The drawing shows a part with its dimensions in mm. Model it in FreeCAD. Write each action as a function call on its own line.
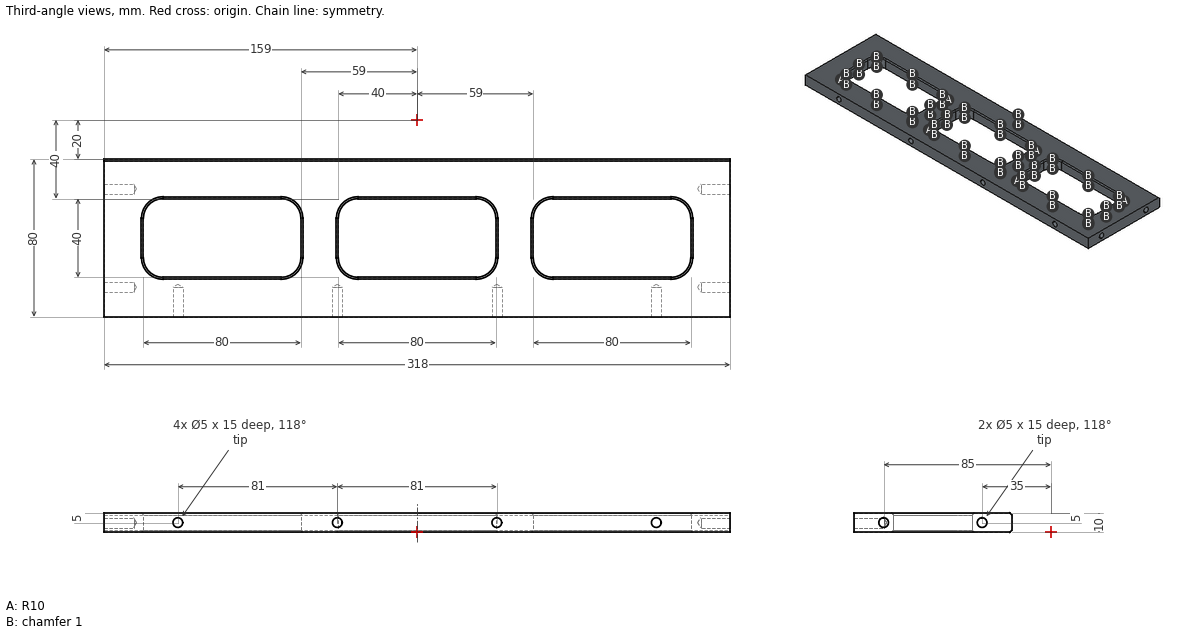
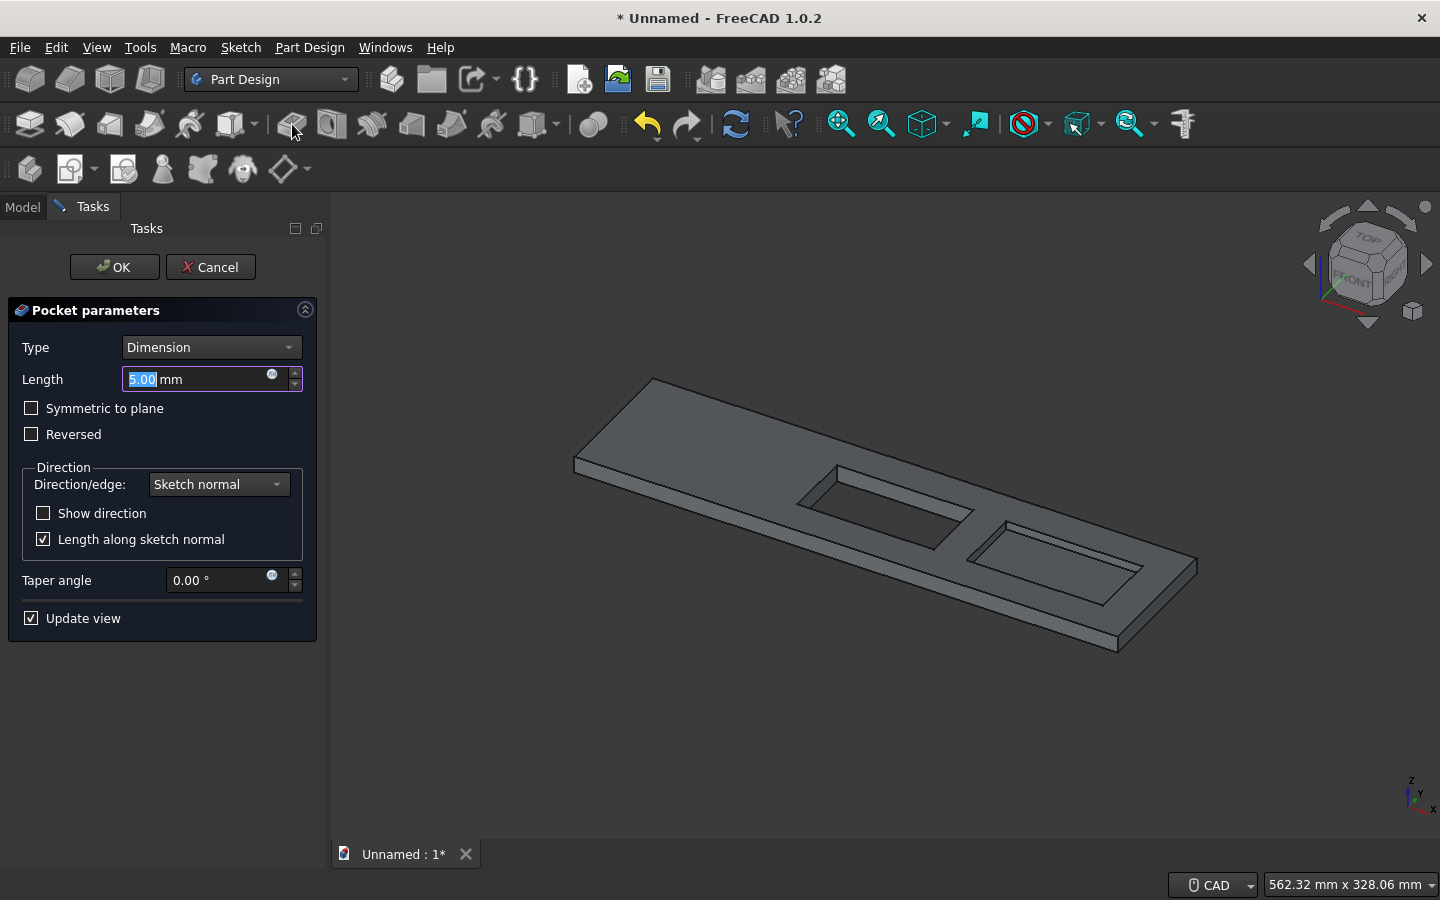
click(212, 348)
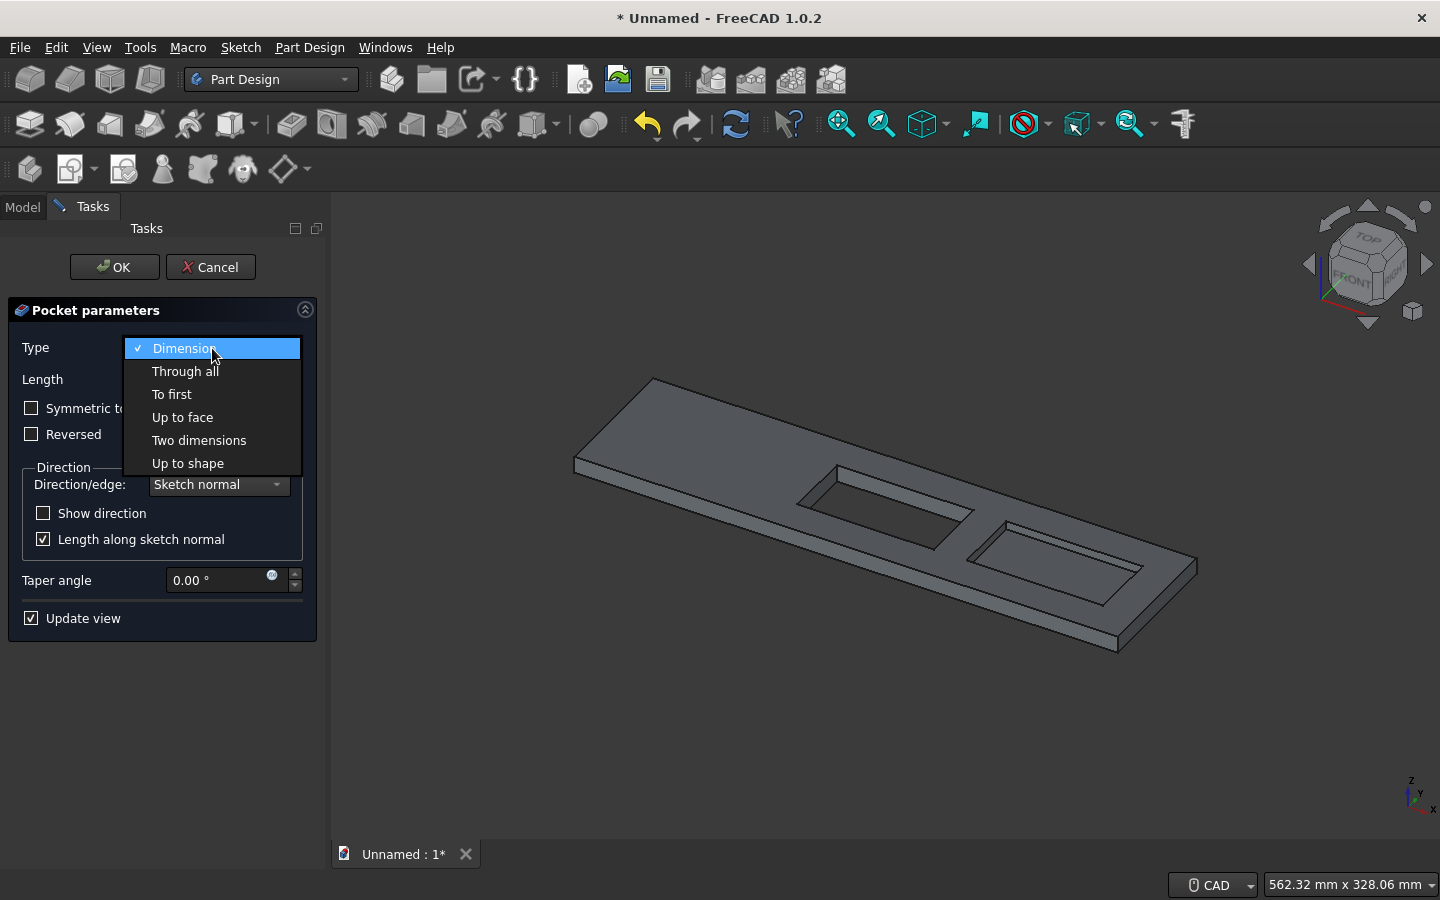
click(212, 372)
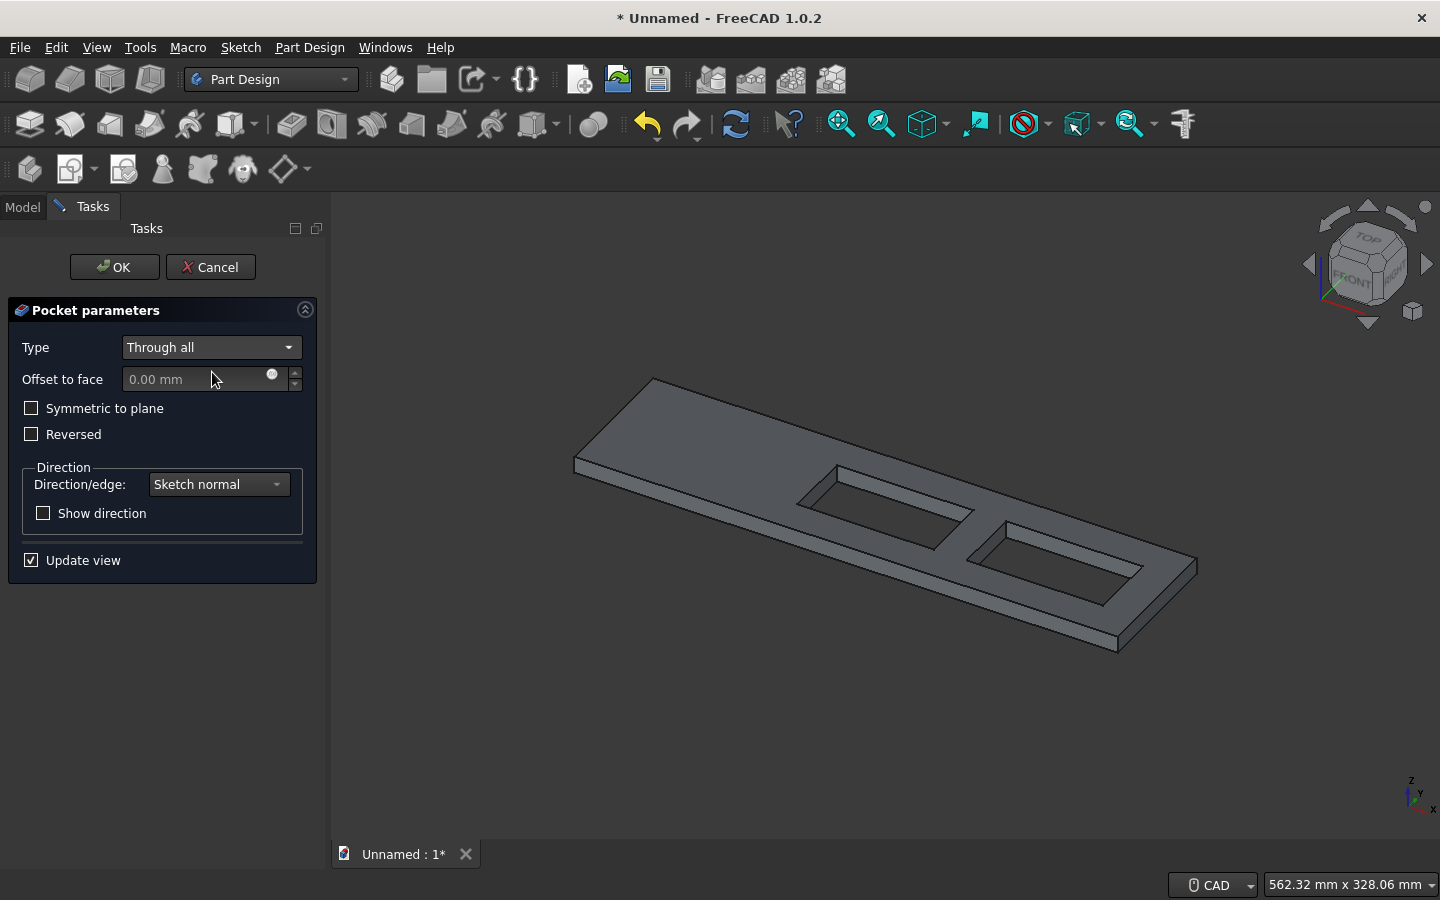
click(115, 267)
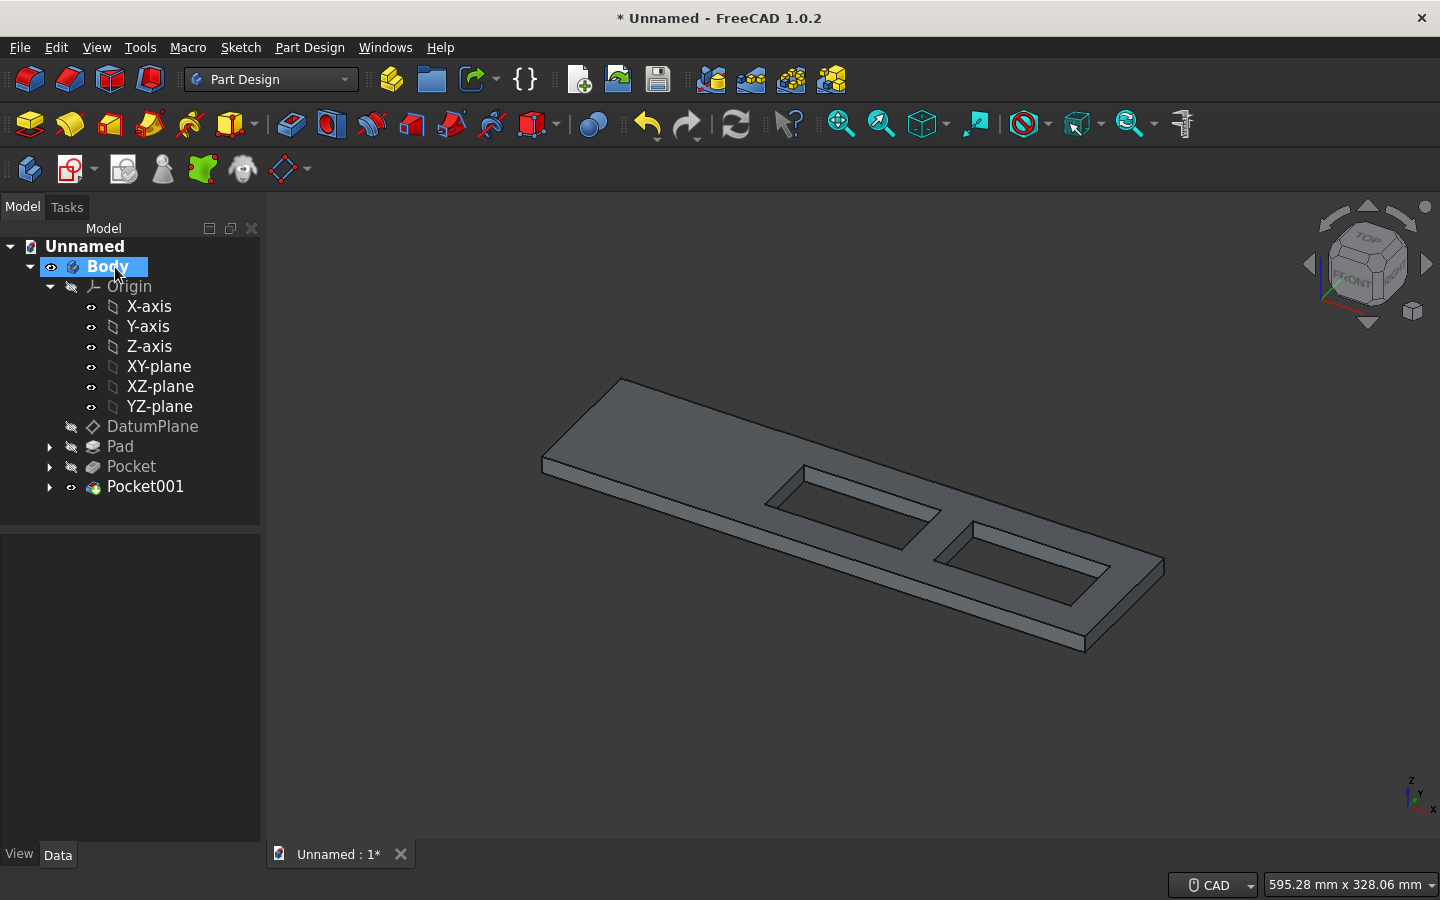
click(70, 170)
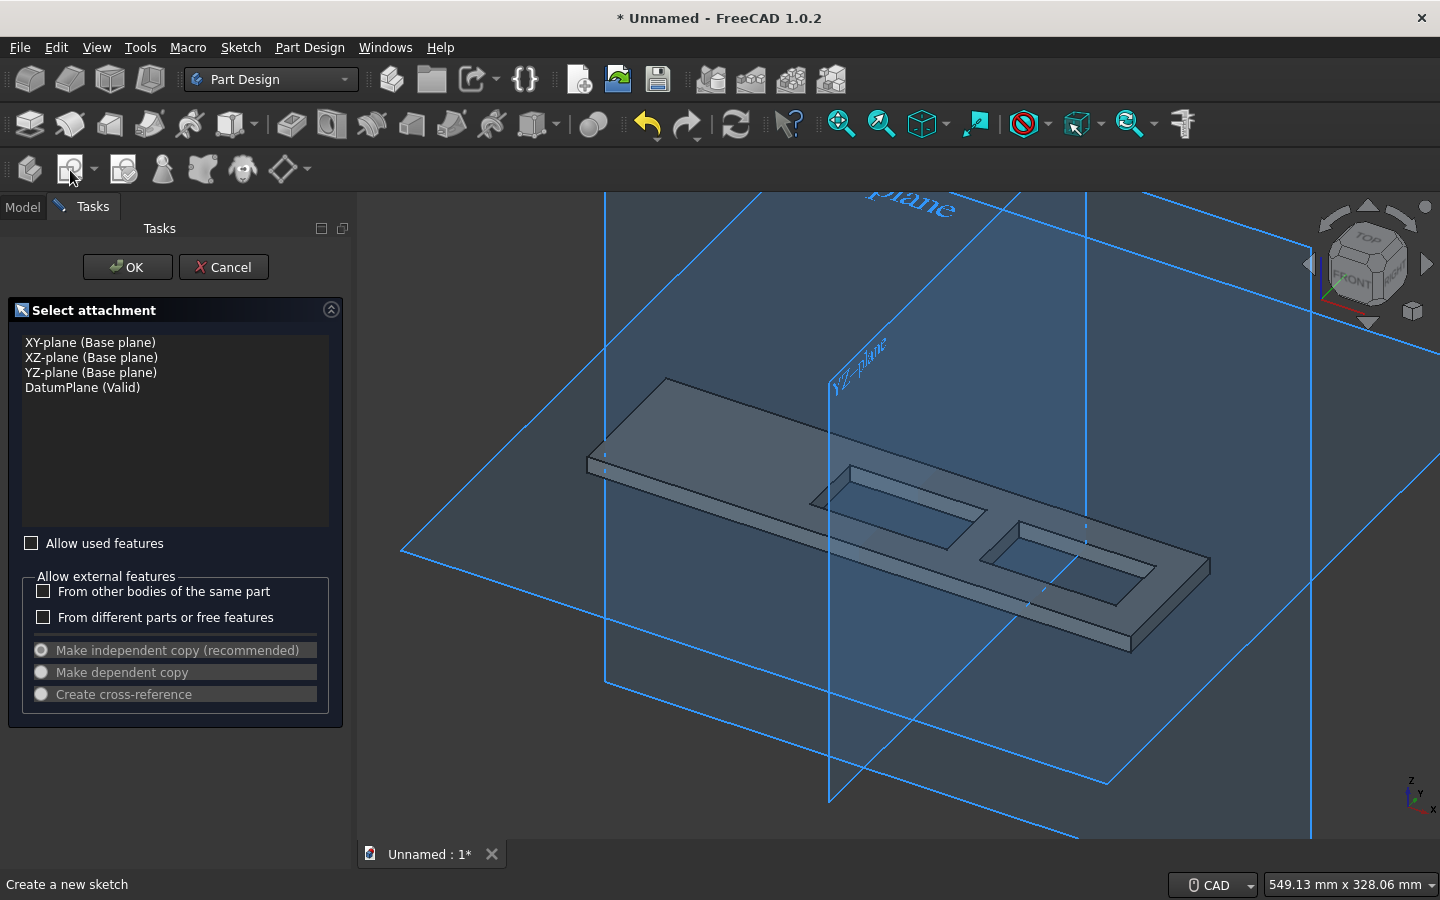
click(82, 342)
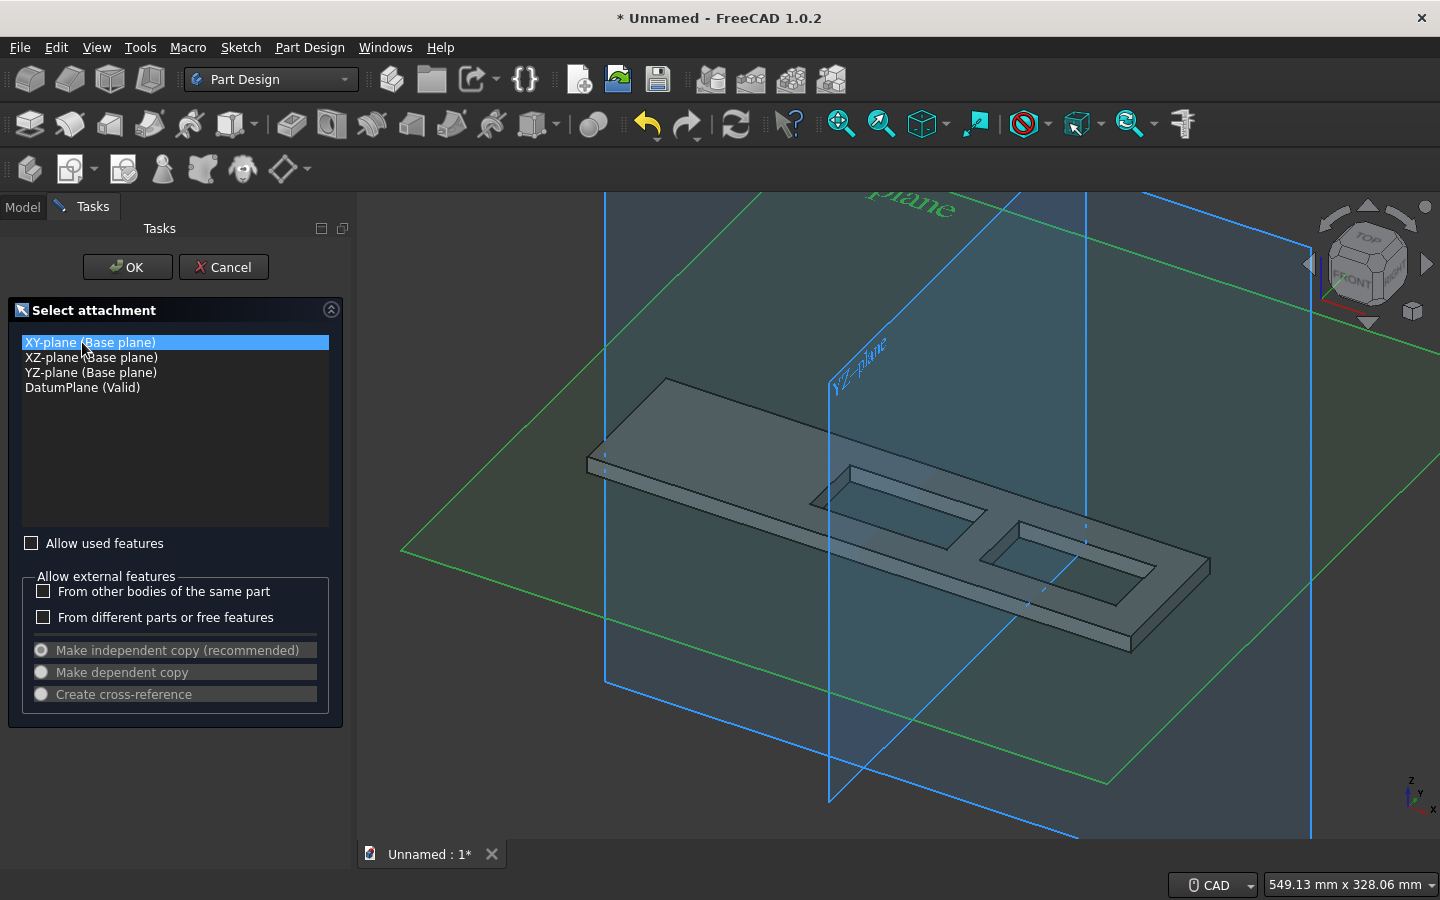
click(128, 267)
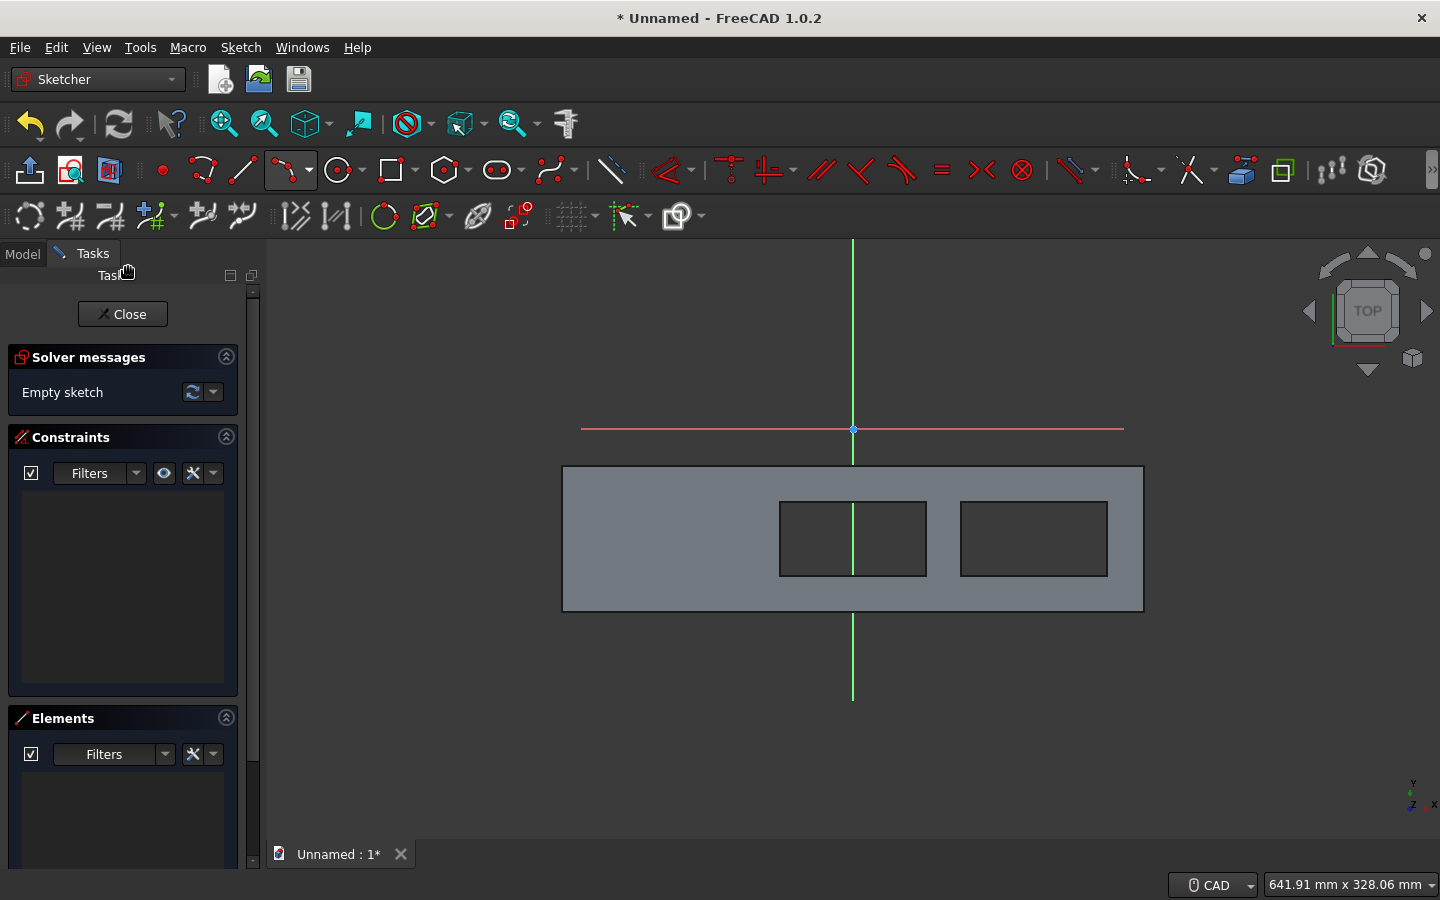
click(110, 170)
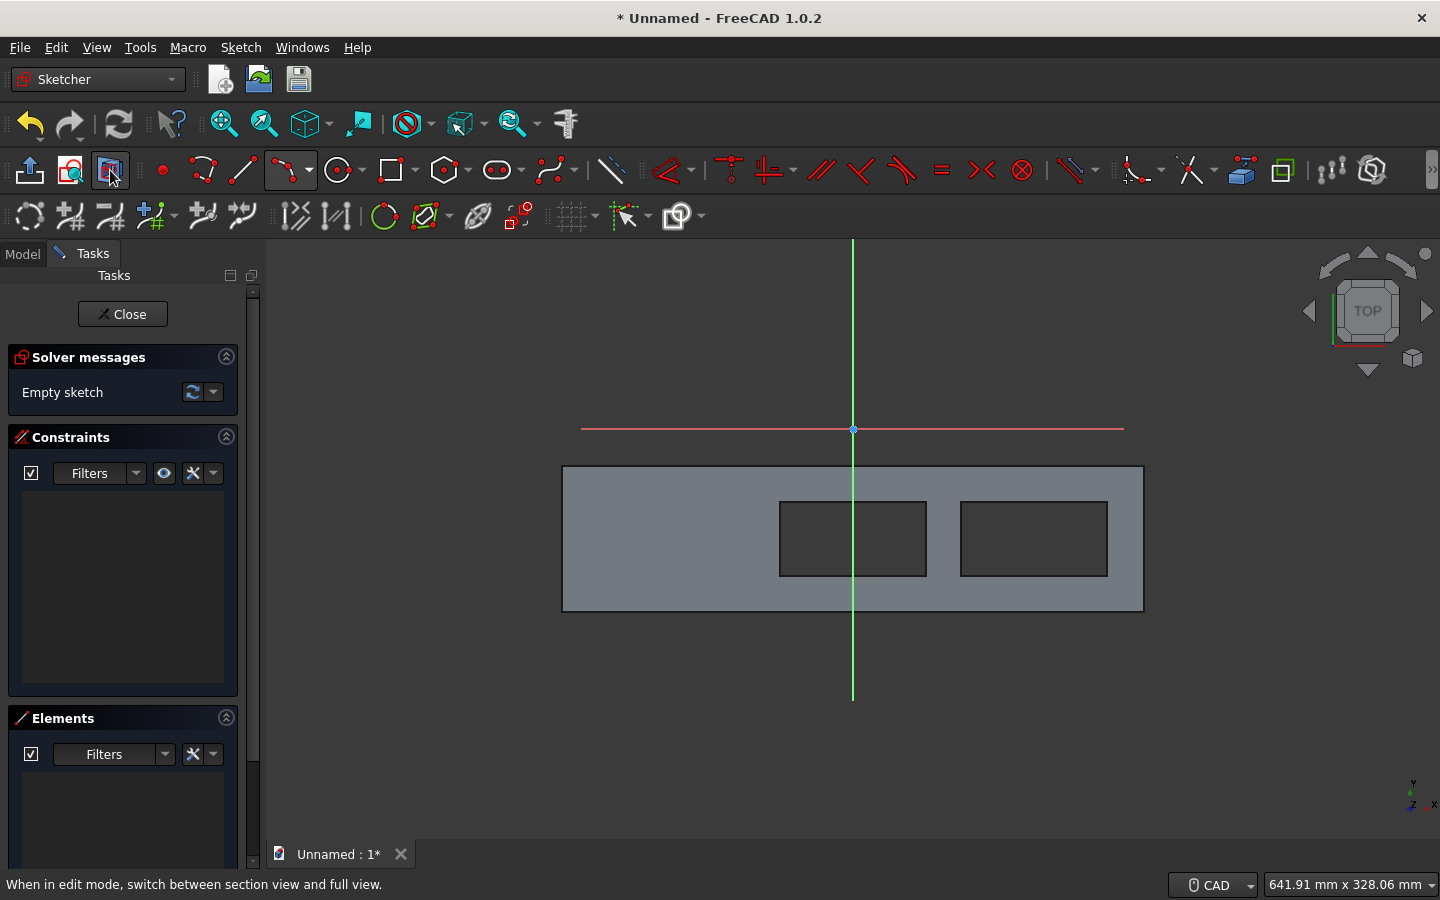
scroll(692, 481, up, 5)